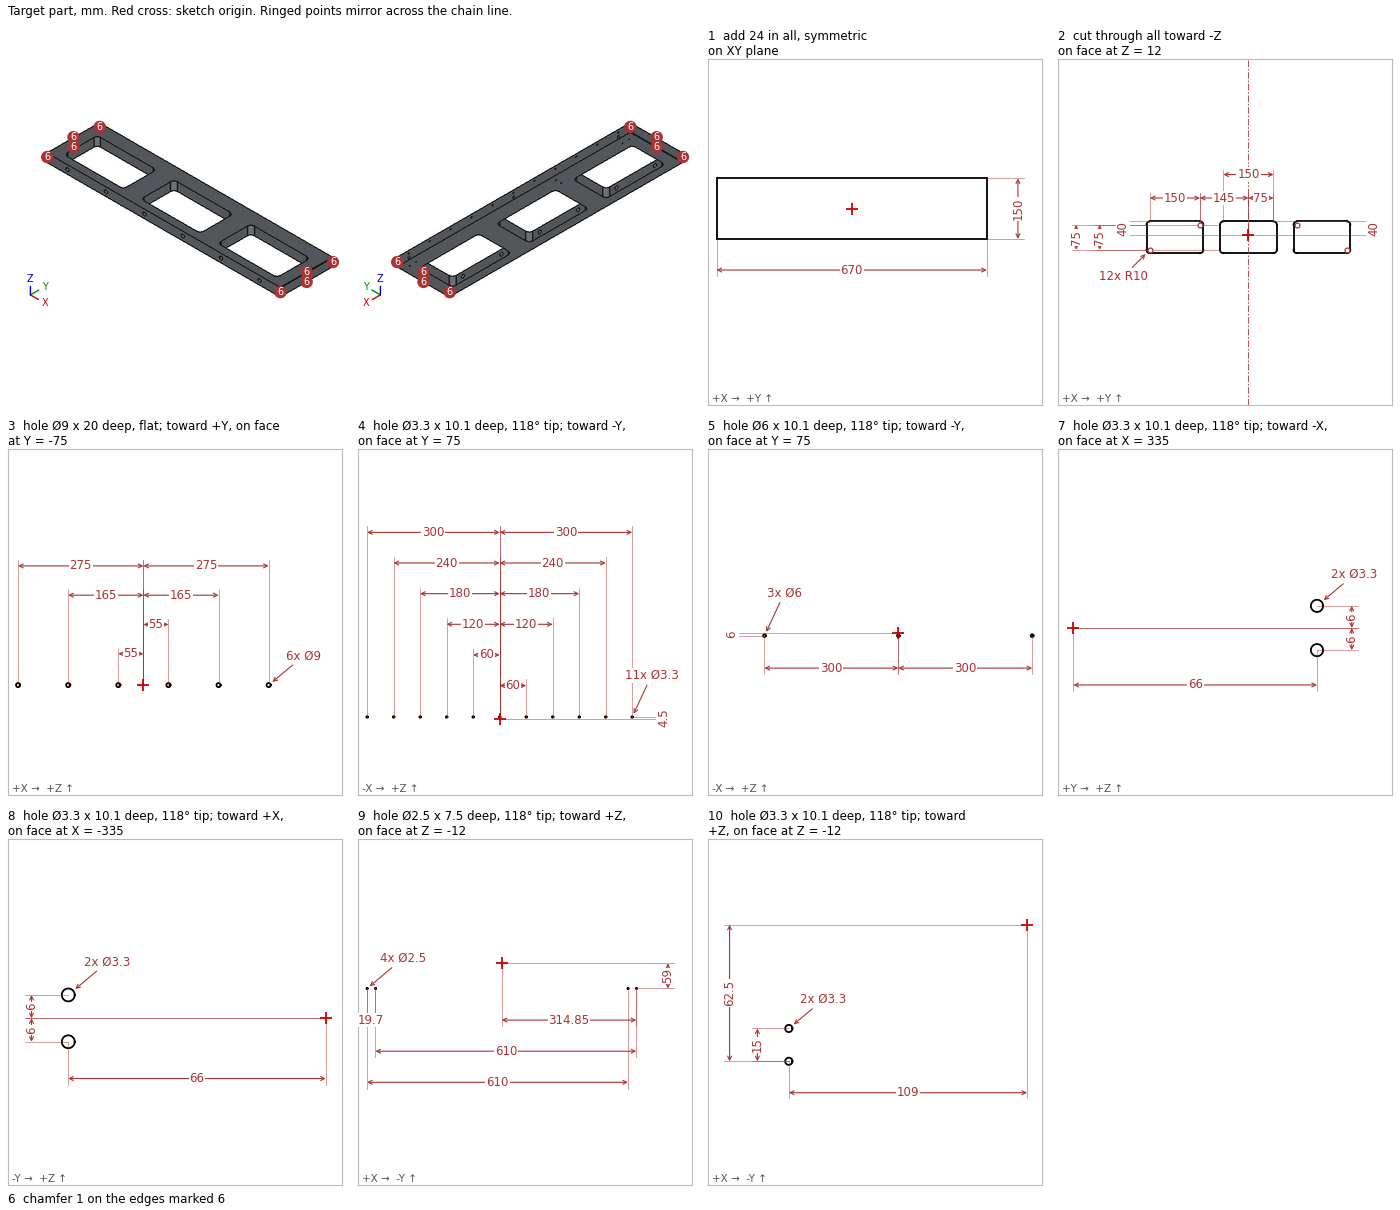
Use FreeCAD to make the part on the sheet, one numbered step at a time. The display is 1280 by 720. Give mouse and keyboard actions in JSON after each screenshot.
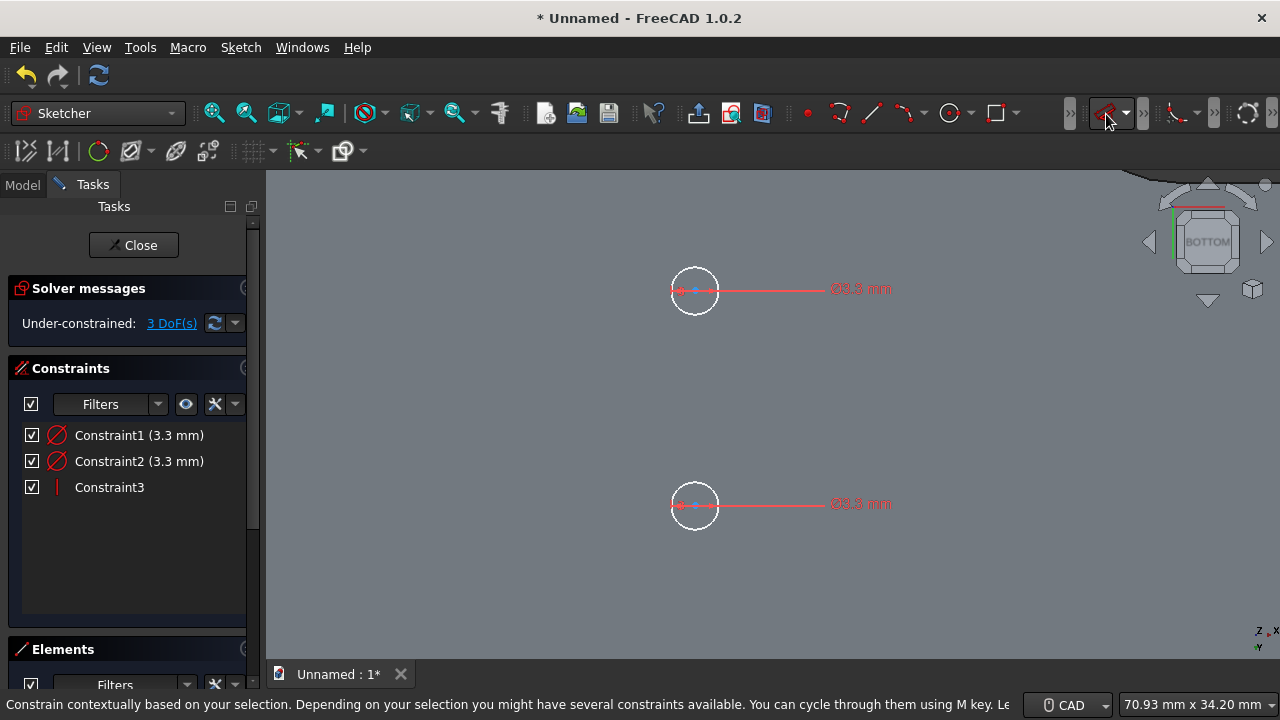
{"action": "left_click", "coordinate": [695, 506]}
{"action": "left_click", "coordinate": [905, 540]}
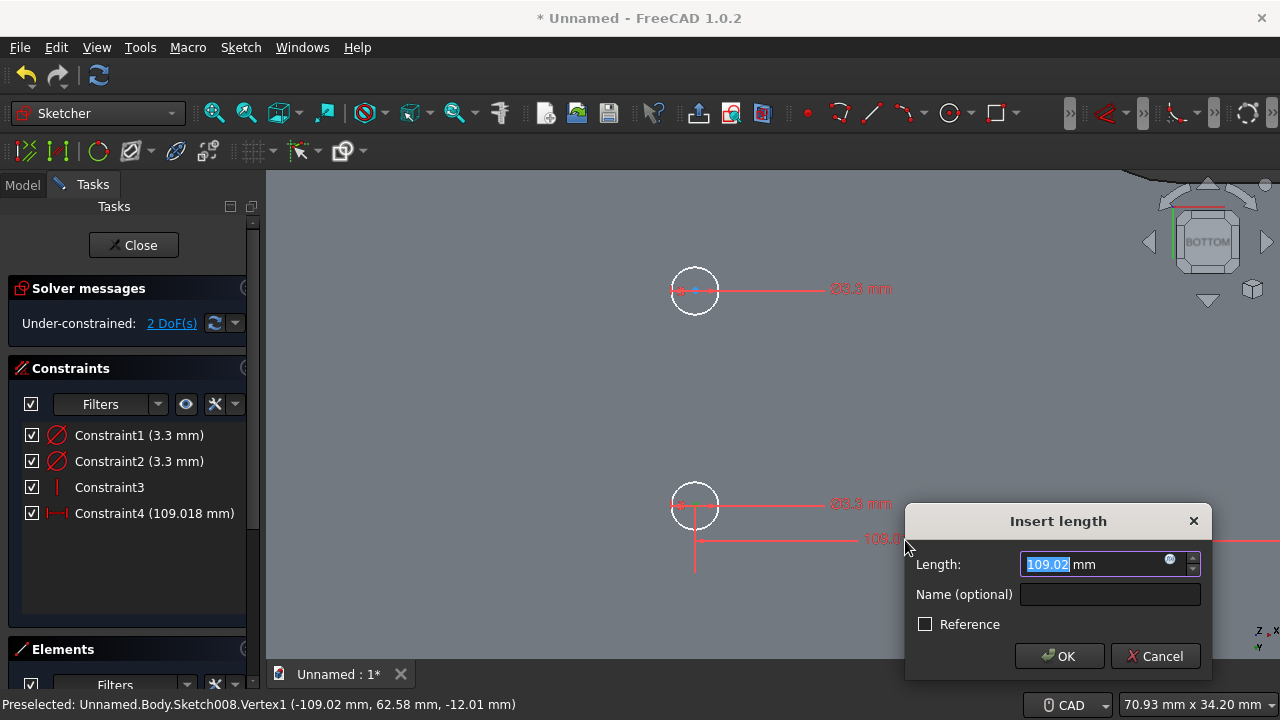
{"action": "type", "text": "109"}
{"action": "key", "text": "Return"}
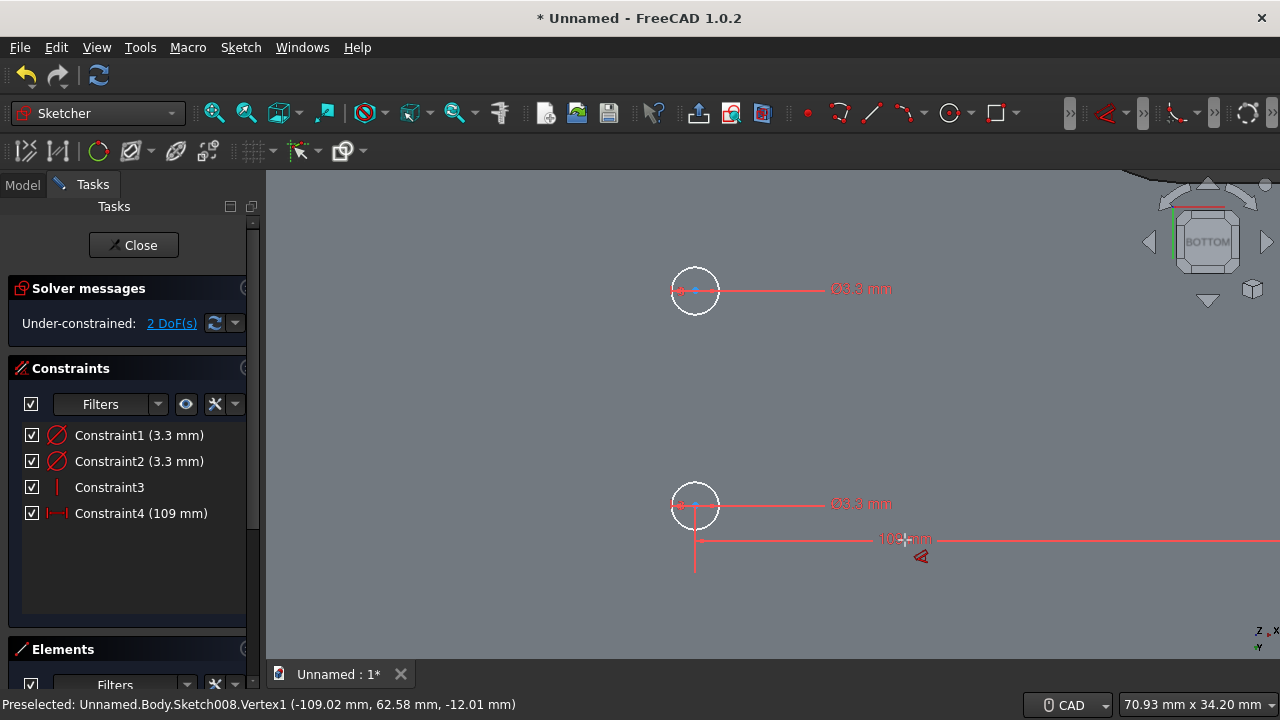
{"action": "left_click", "coordinate": [695, 506]}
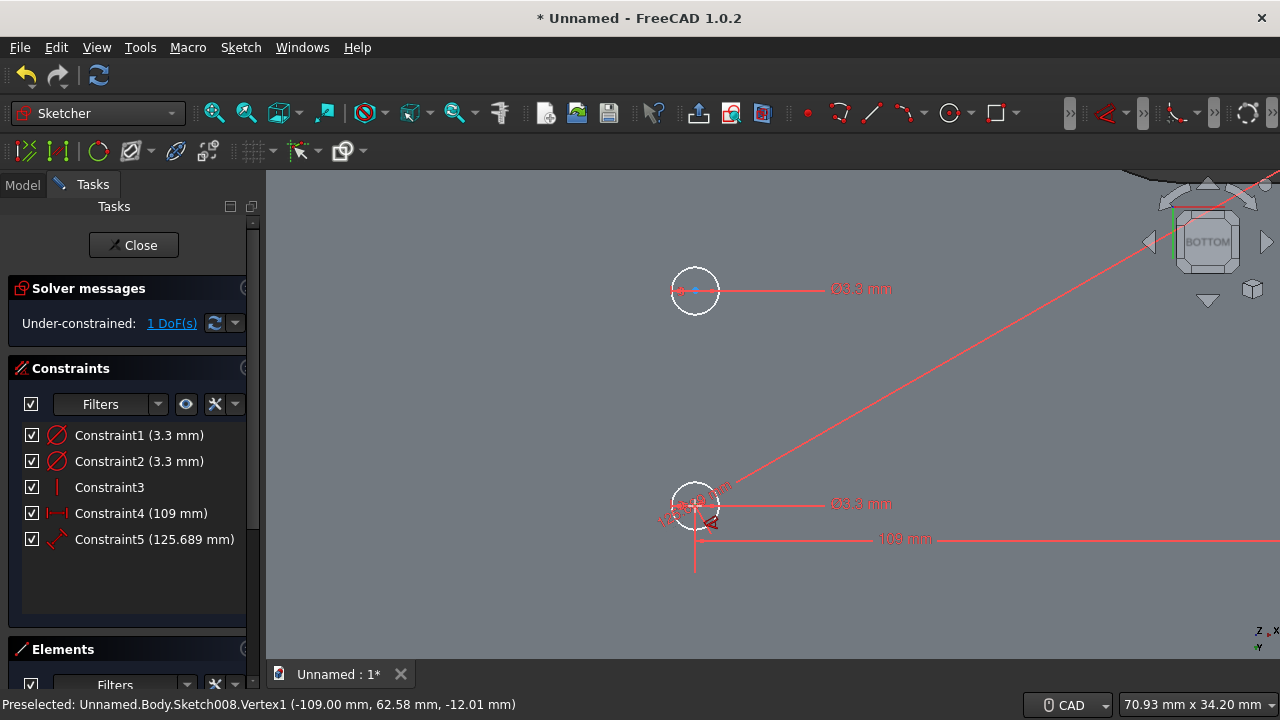
{"action": "left_click", "coordinate": [695, 291]}
{"action": "left_click", "coordinate": [729, 399]}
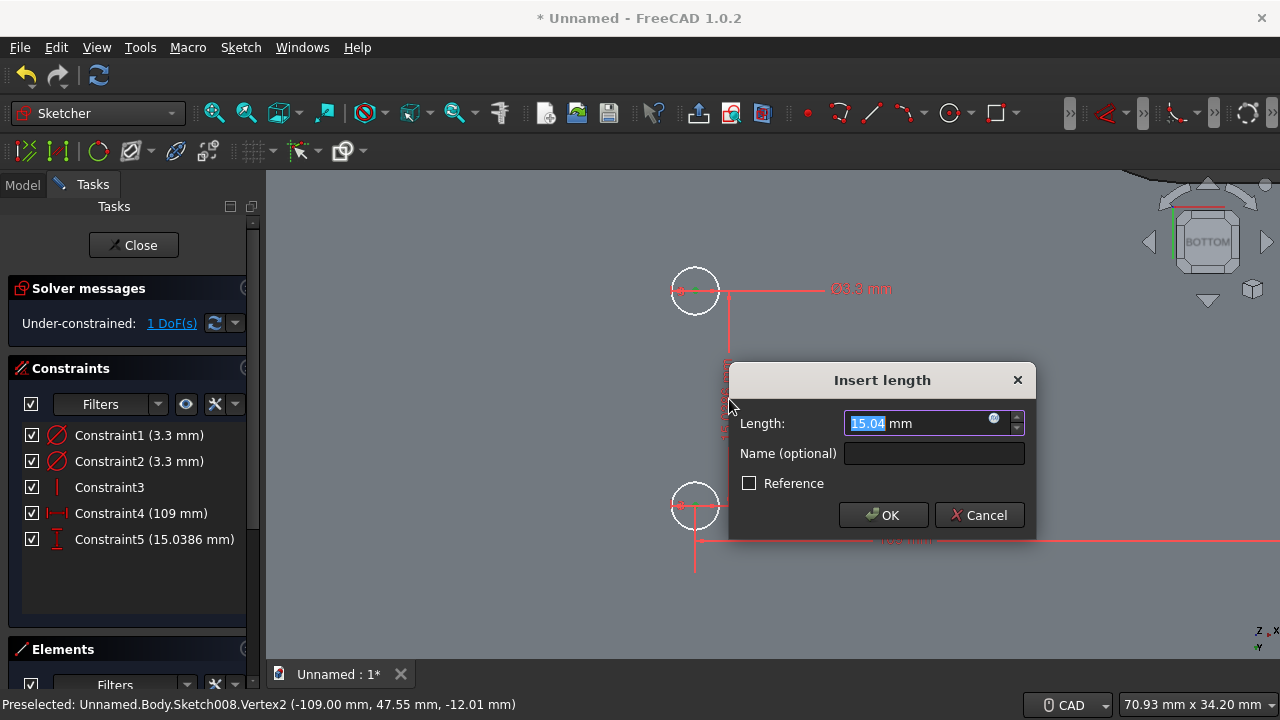
{"action": "type", "text": "15"}
{"action": "key", "text": "Return"}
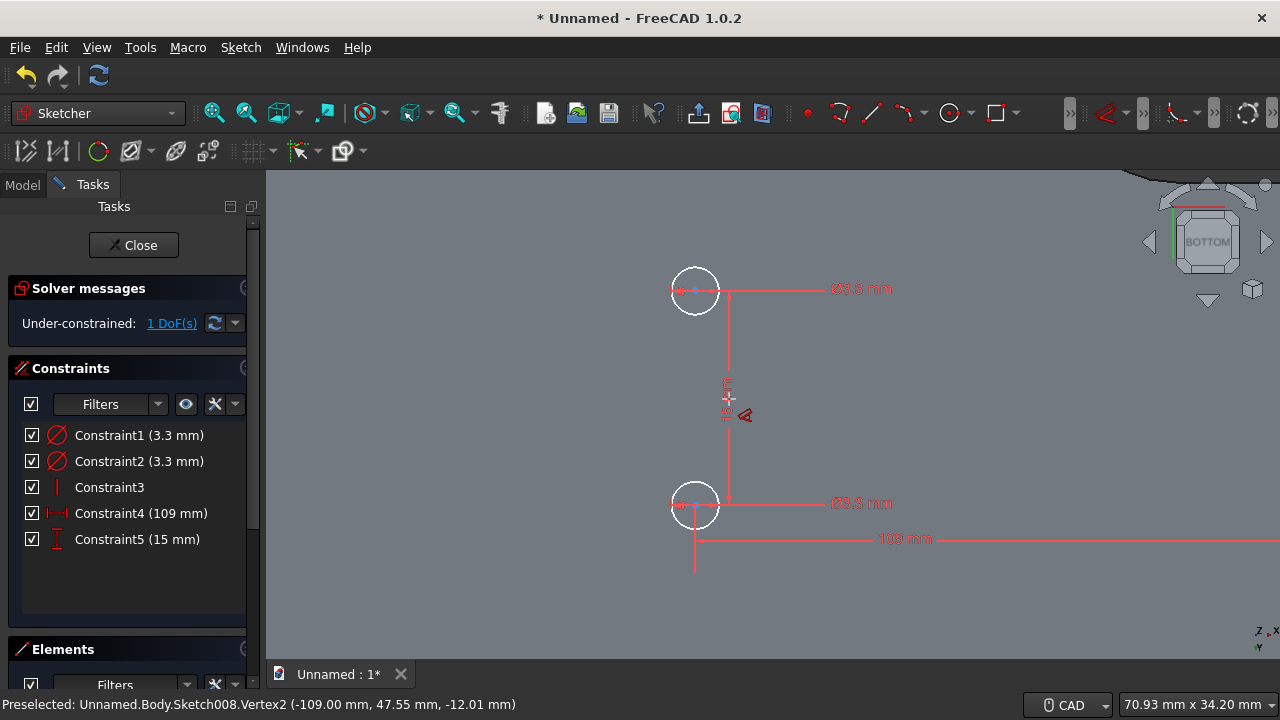
{"action": "left_click", "coordinate": [695, 505]}
{"action": "left_click", "coordinate": [661, 352]}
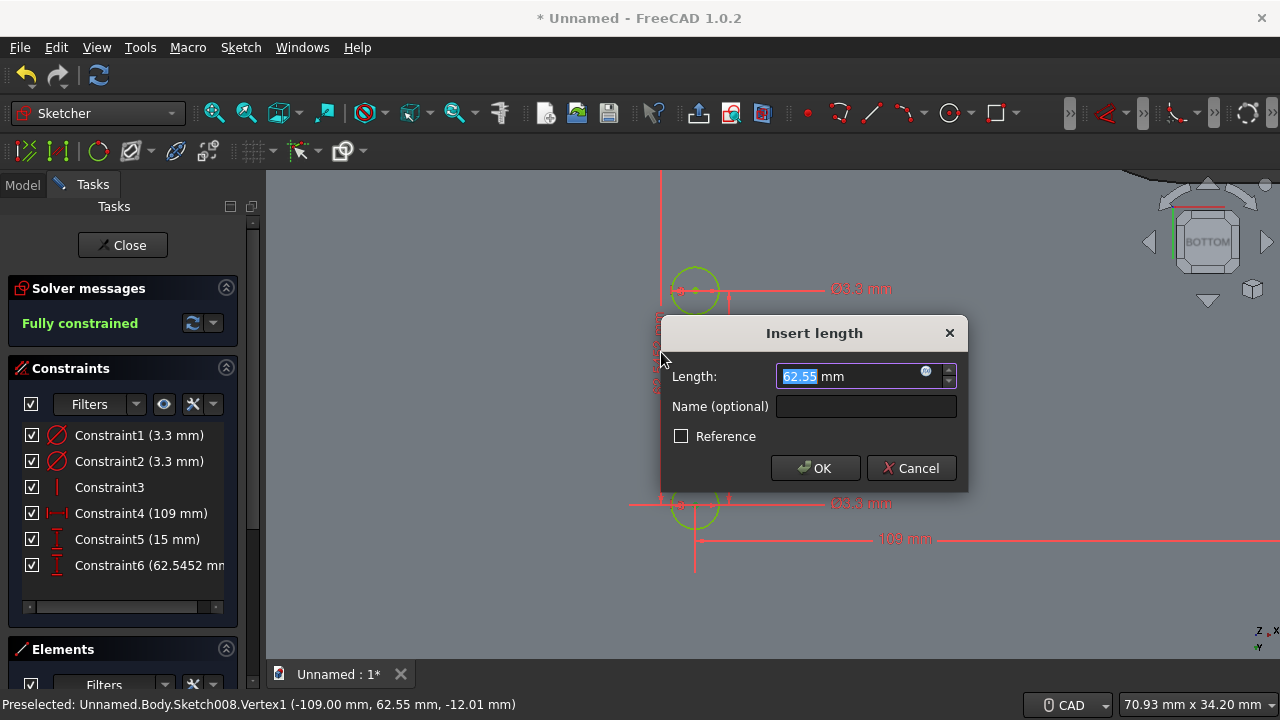
{"action": "type", "text": "62.5"}
{"action": "key", "text": "Return"}
{"action": "key", "text": "Escape"}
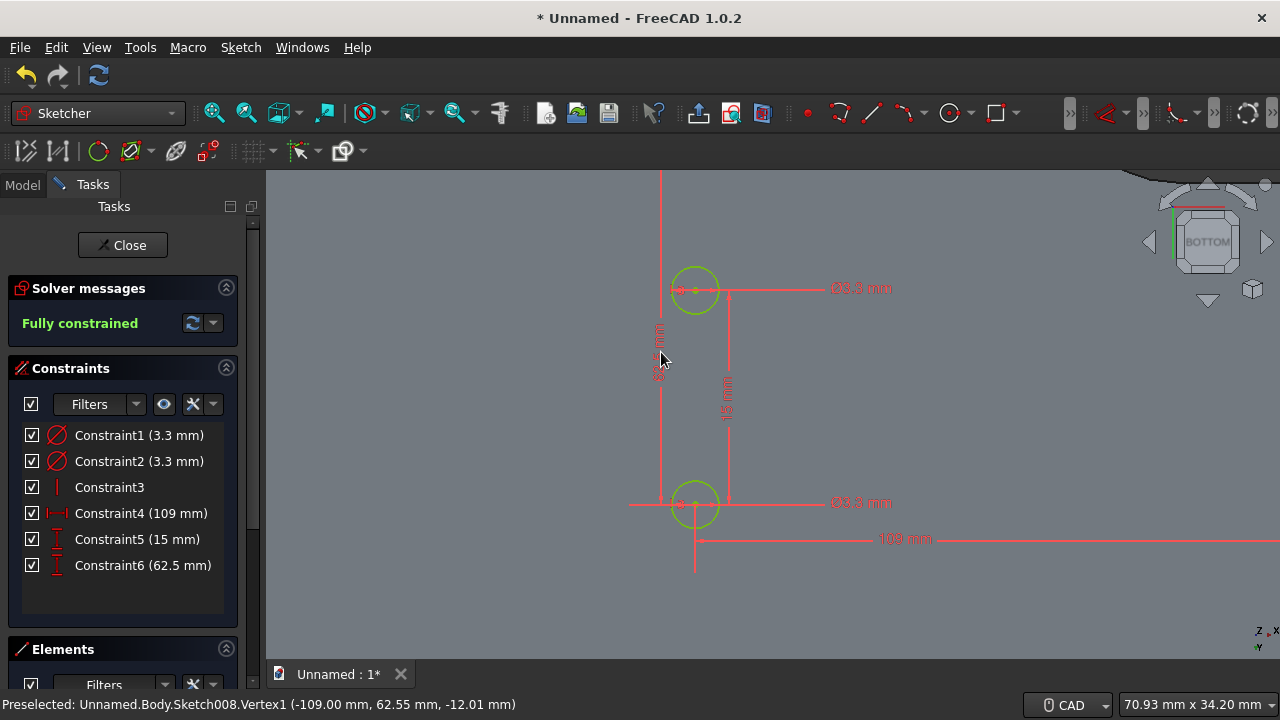
{"action": "left_click", "coordinate": [123, 245]}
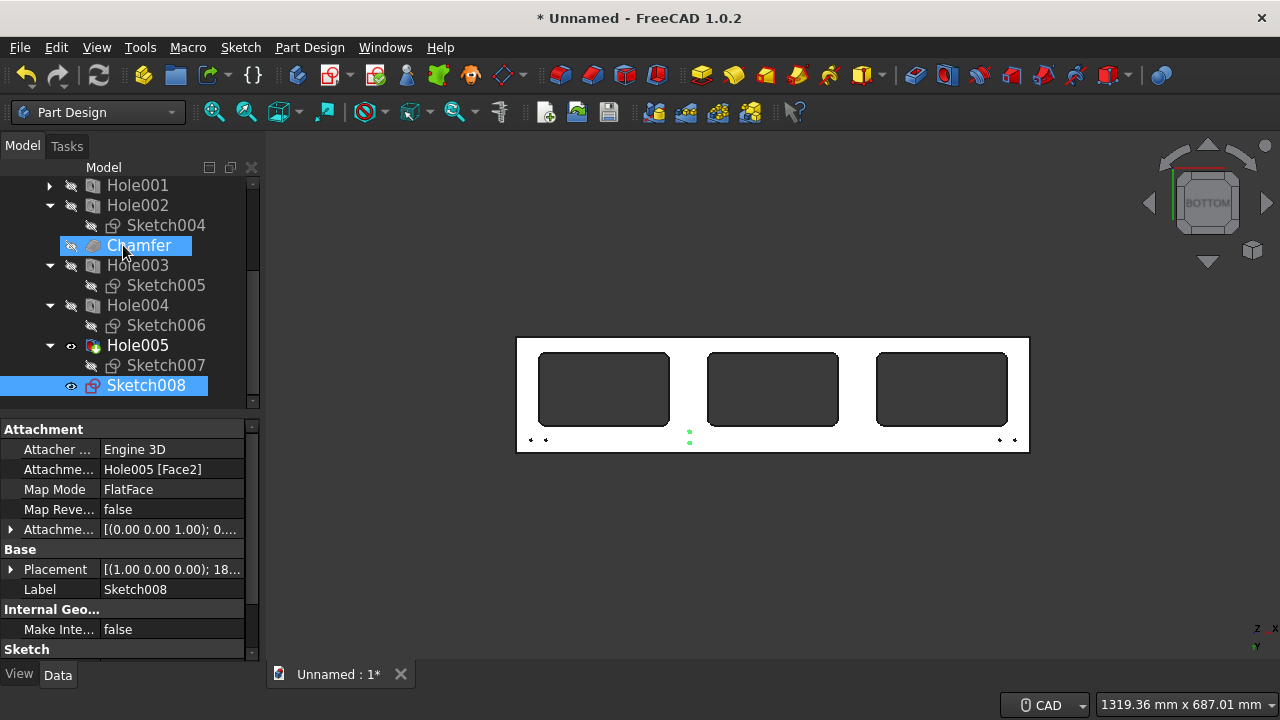
{"action": "left_click", "coordinate": [948, 76]}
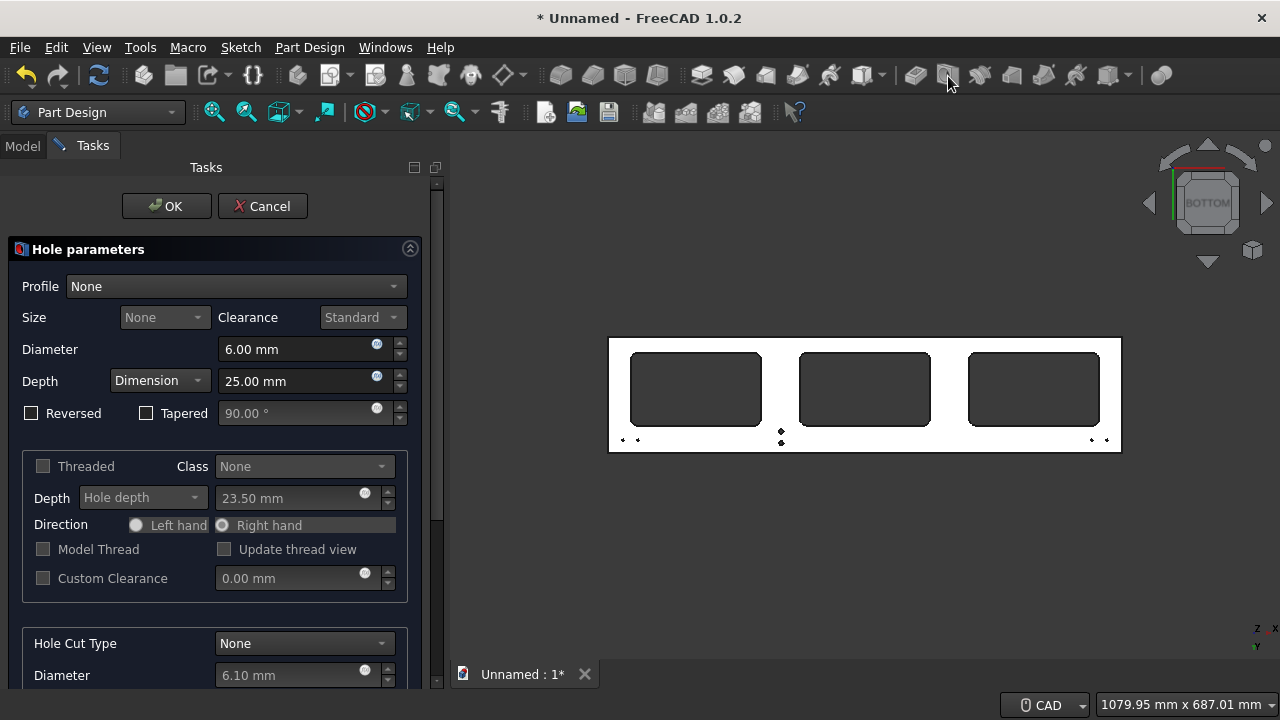
{"action": "triple_click", "coordinate": [305, 349]}